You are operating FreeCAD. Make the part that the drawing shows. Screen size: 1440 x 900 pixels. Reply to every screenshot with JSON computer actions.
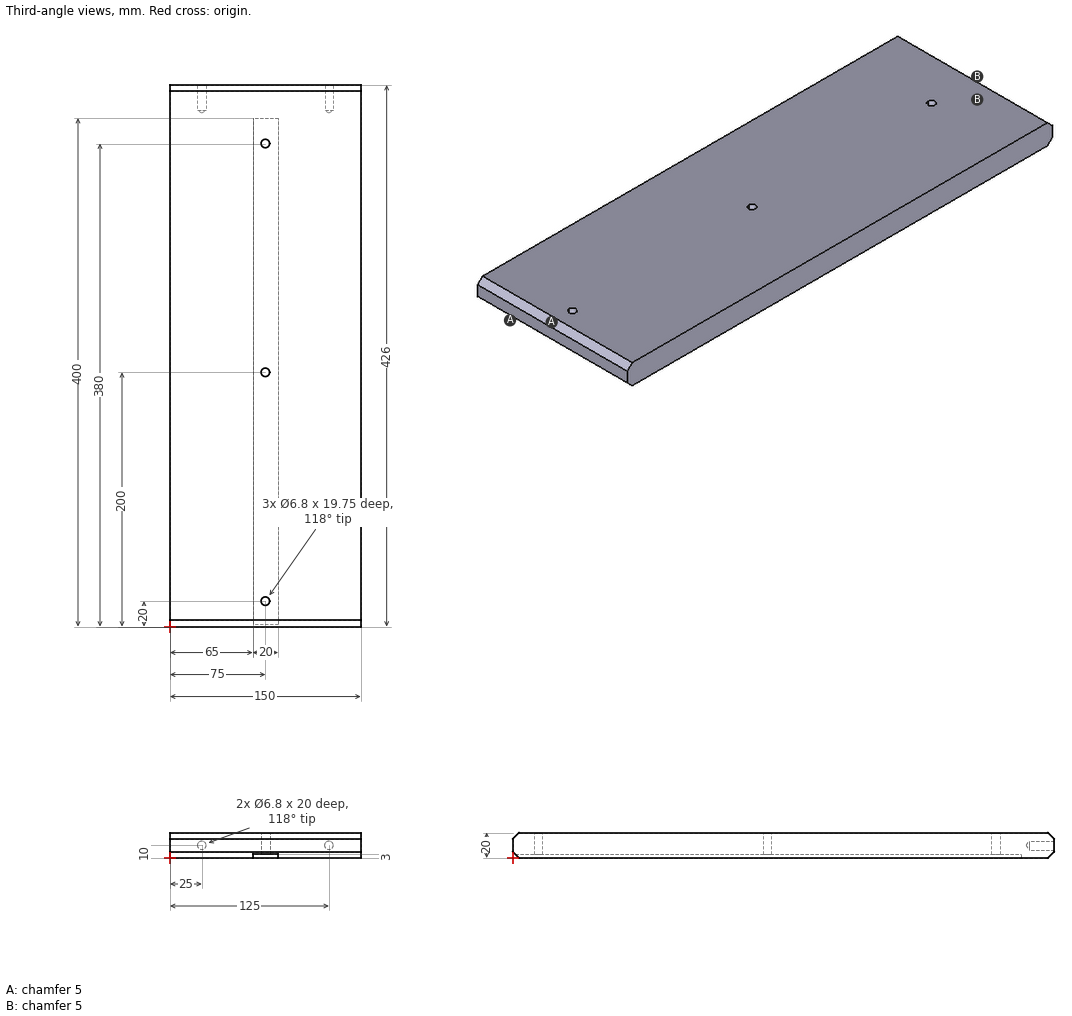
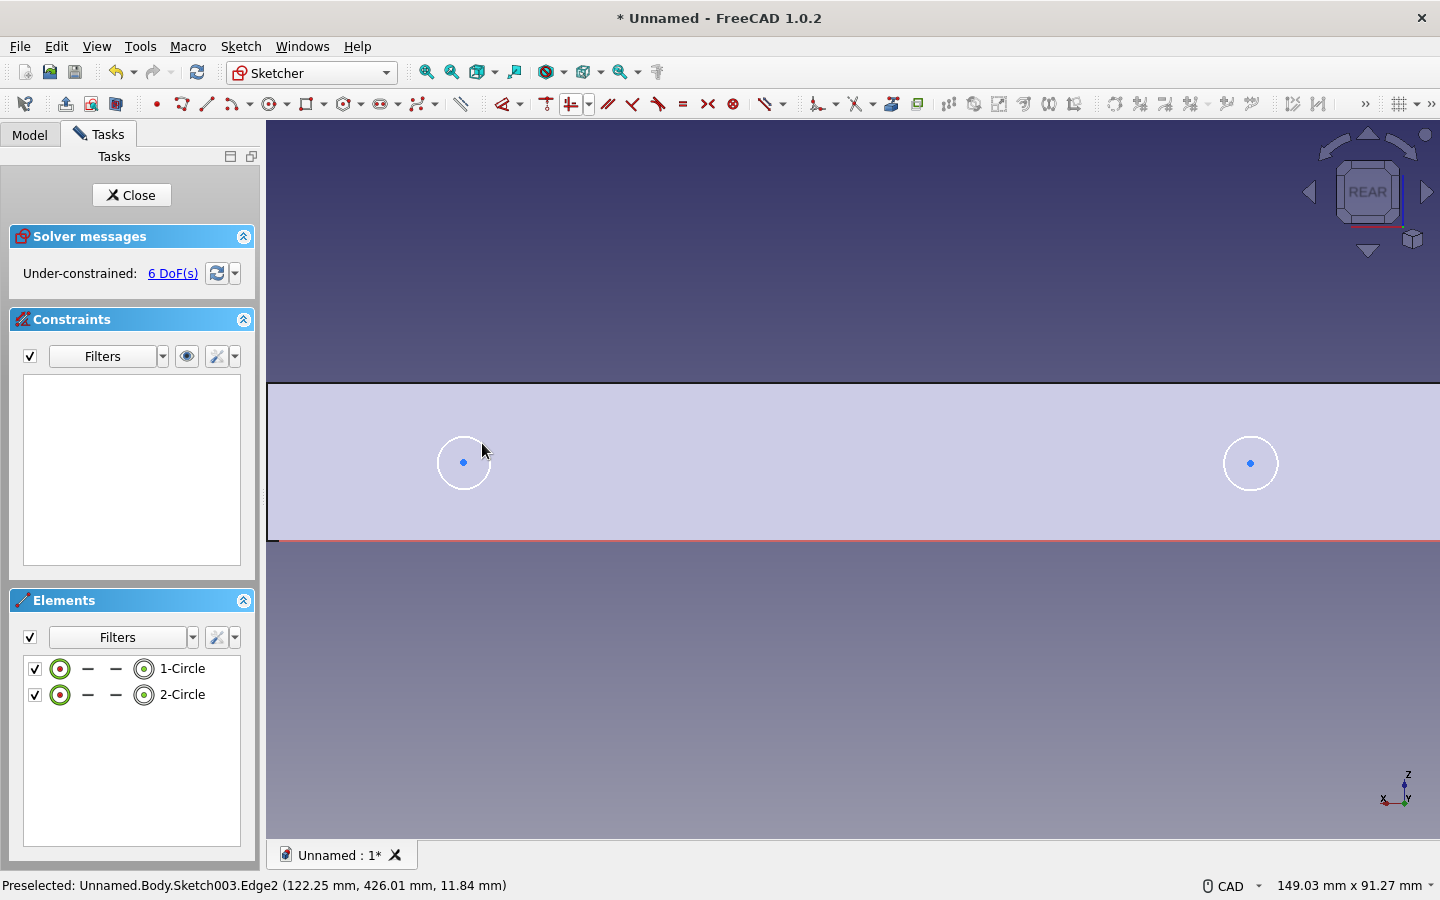
{"action": "left_click", "coordinate": [1270, 444]}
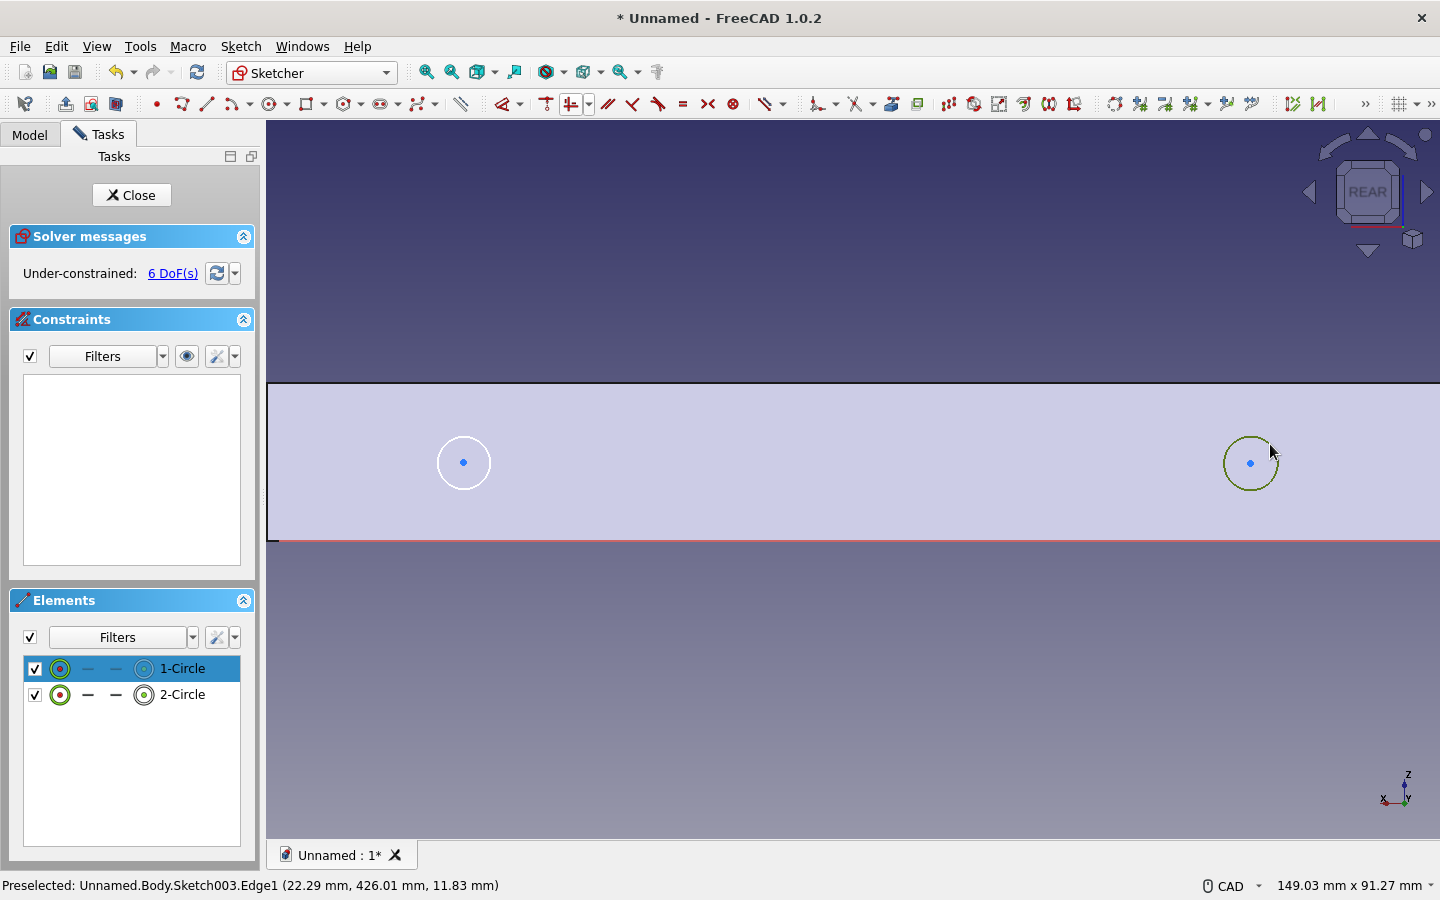
{"action": "left_click", "coordinate": [482, 444]}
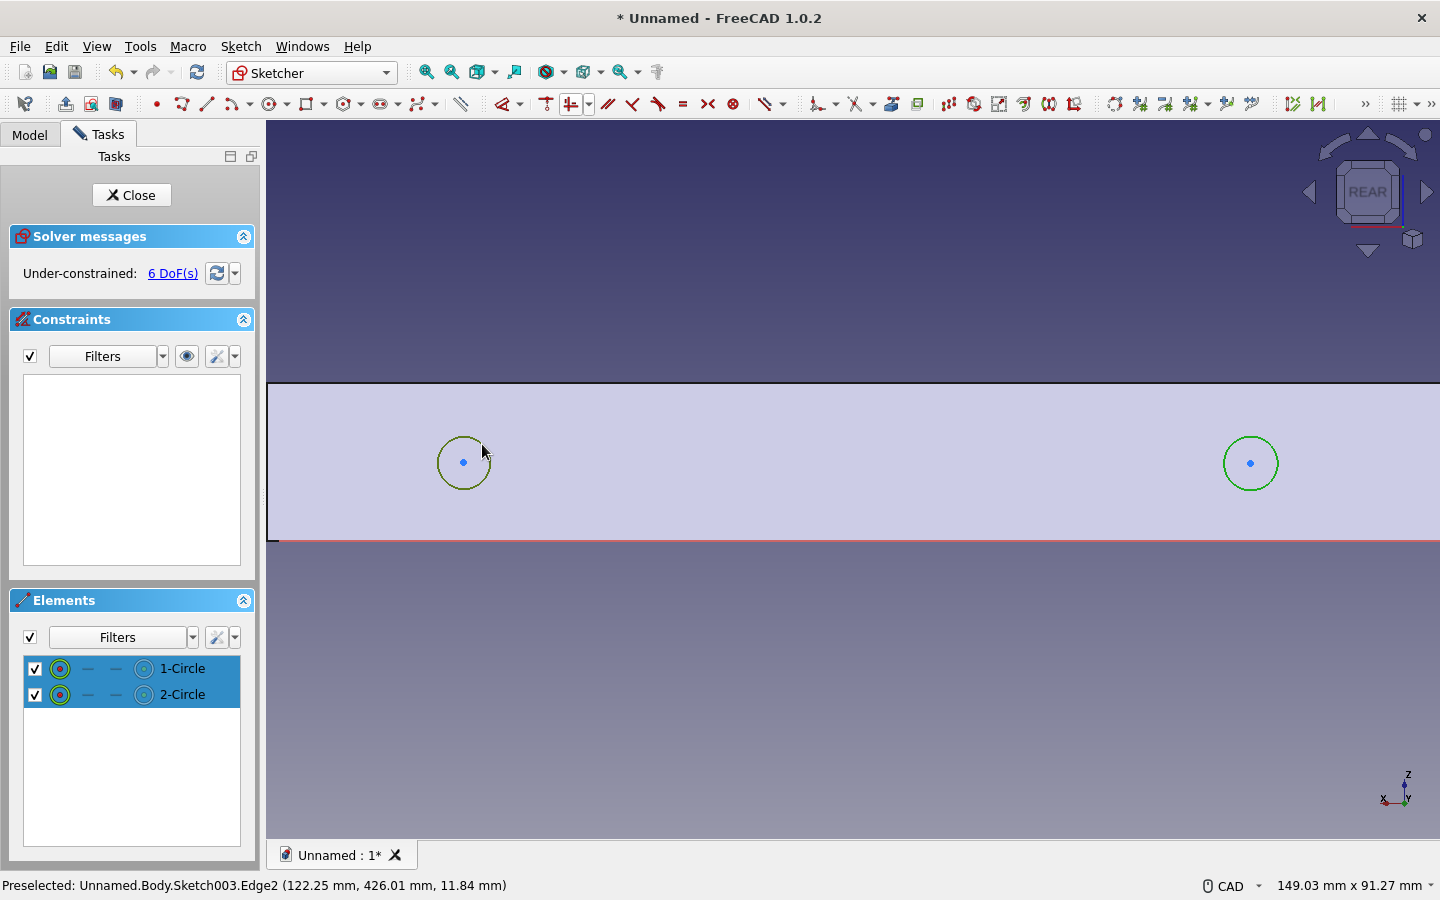
{"action": "left_click", "coordinate": [683, 104]}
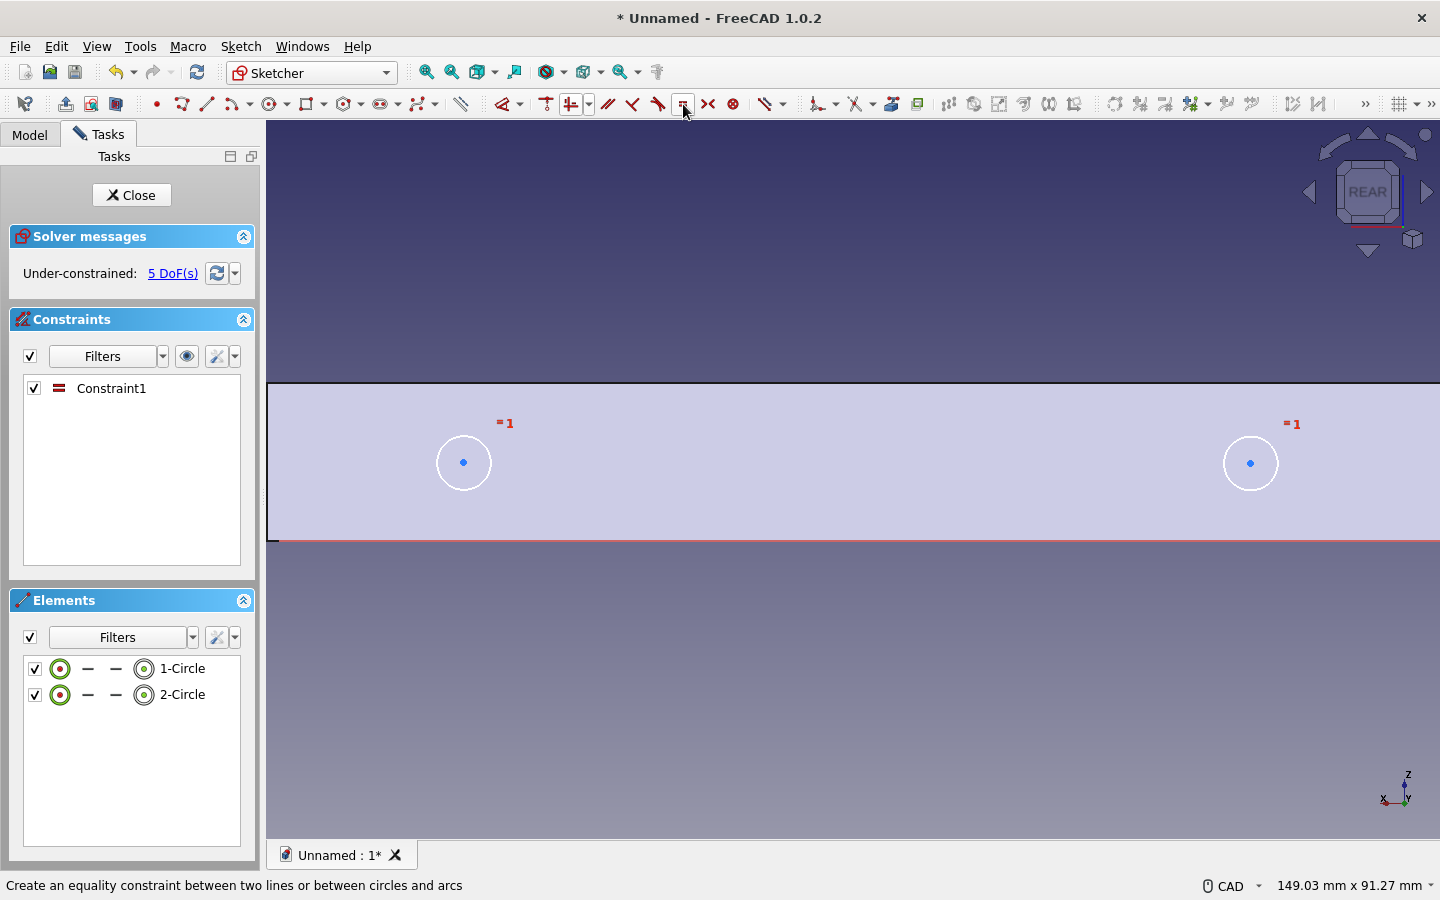
{"action": "left_click", "coordinate": [1251, 463]}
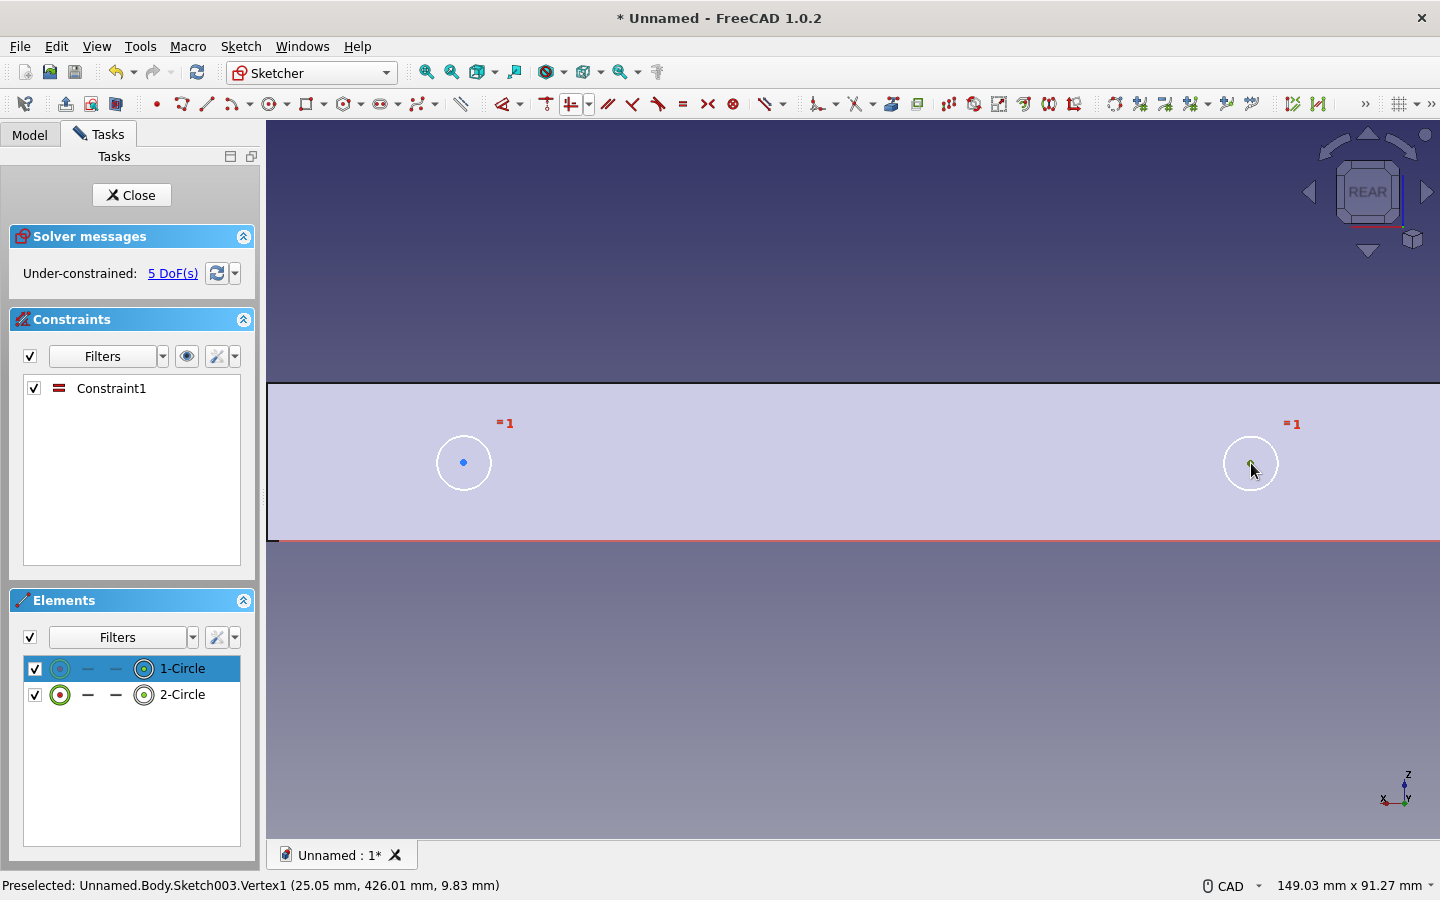
{"action": "left_click", "coordinate": [464, 463]}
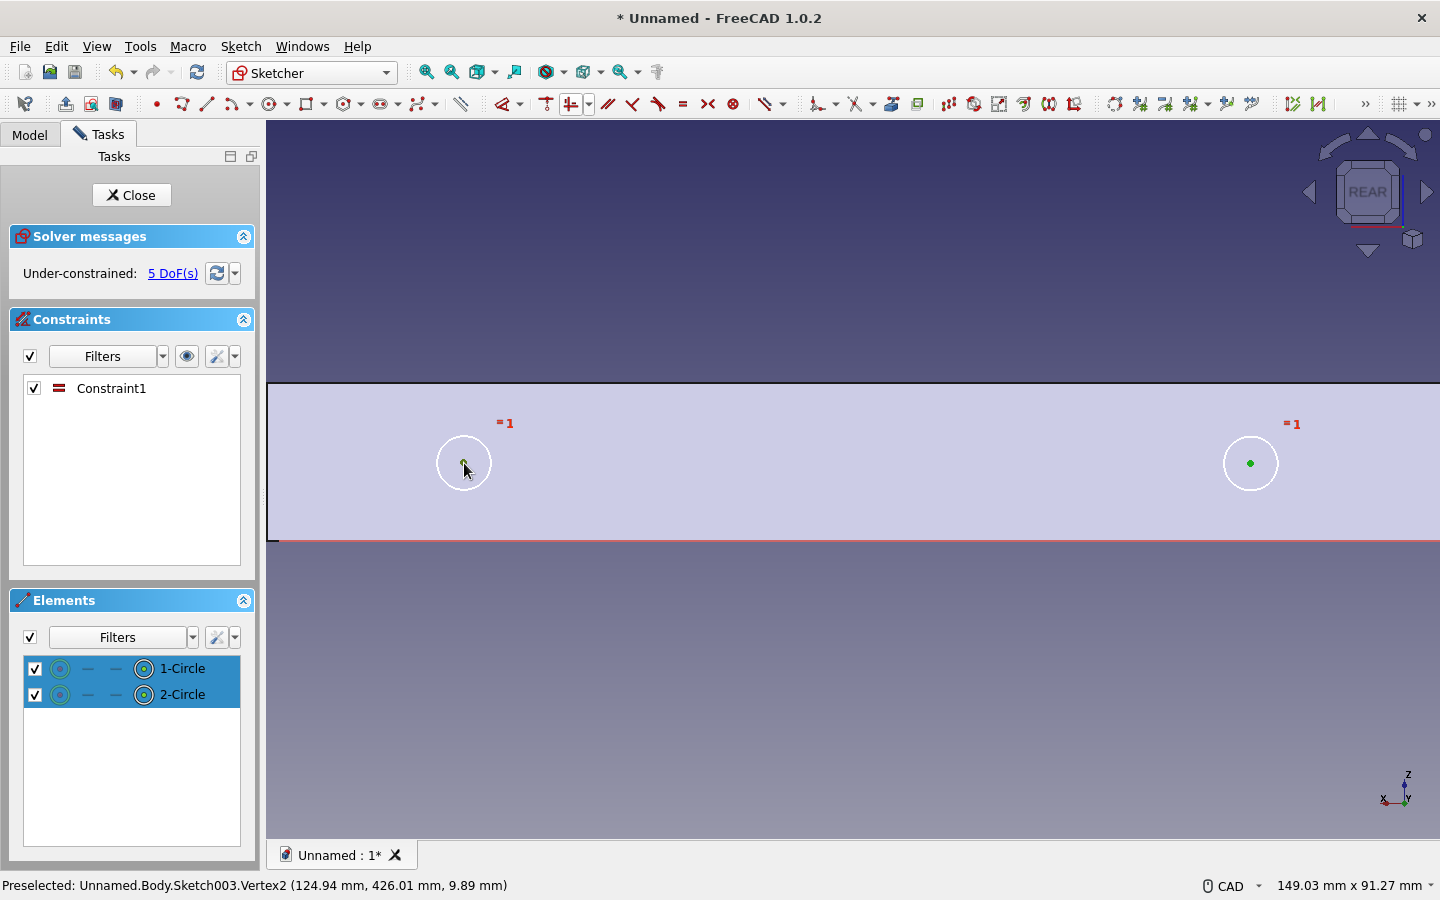
{"action": "left_click", "coordinate": [588, 104]}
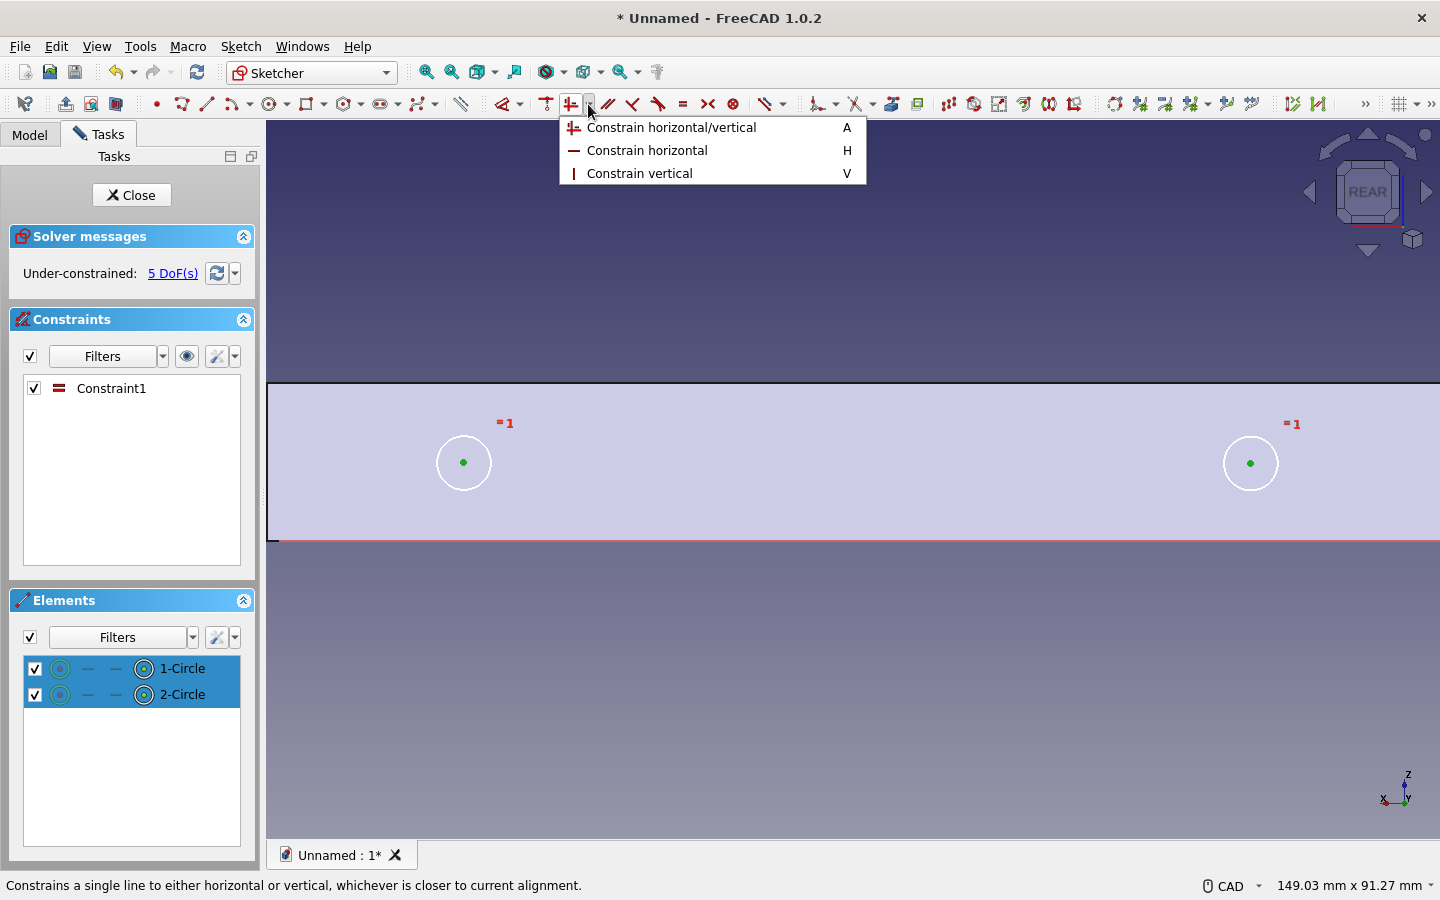
{"action": "left_click", "coordinate": [713, 150]}